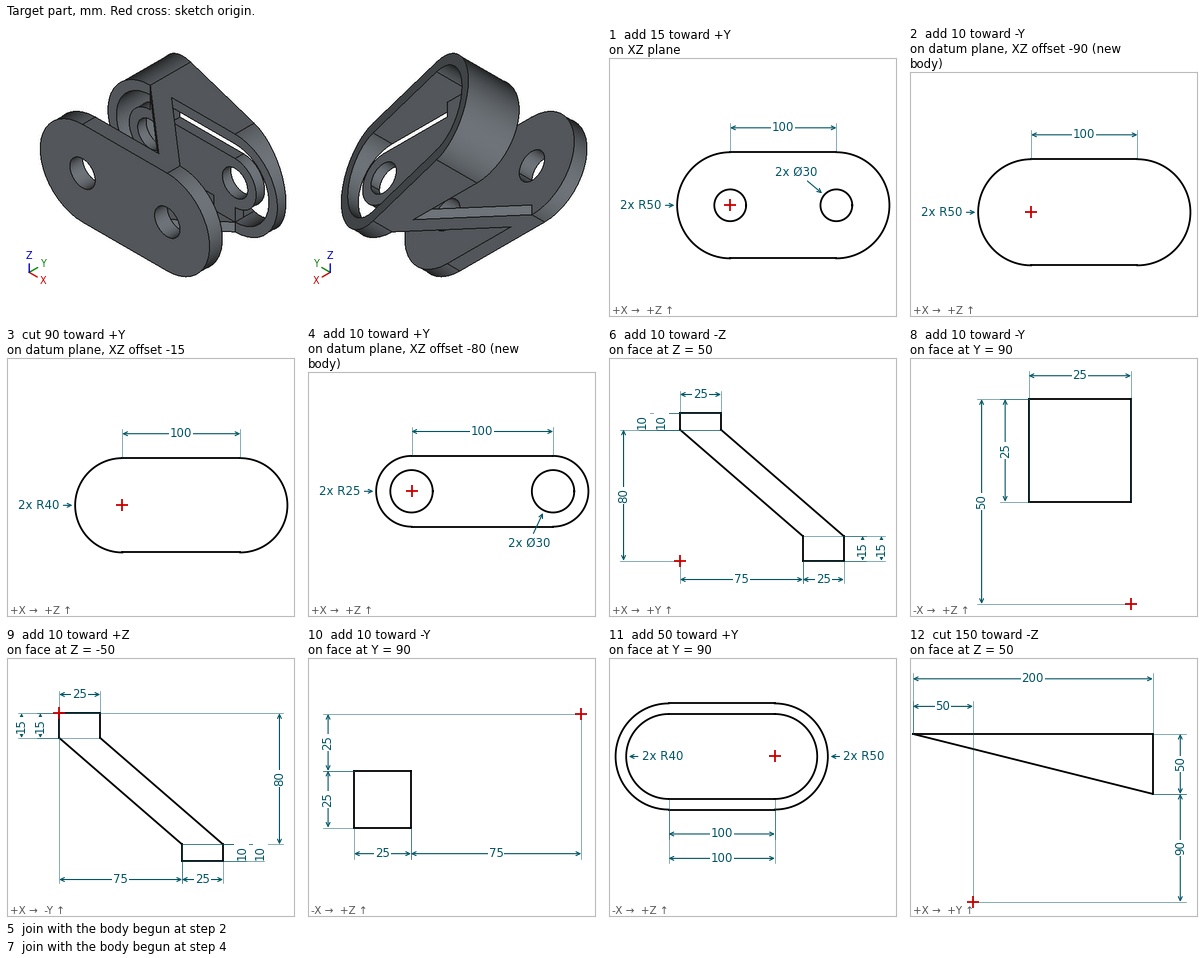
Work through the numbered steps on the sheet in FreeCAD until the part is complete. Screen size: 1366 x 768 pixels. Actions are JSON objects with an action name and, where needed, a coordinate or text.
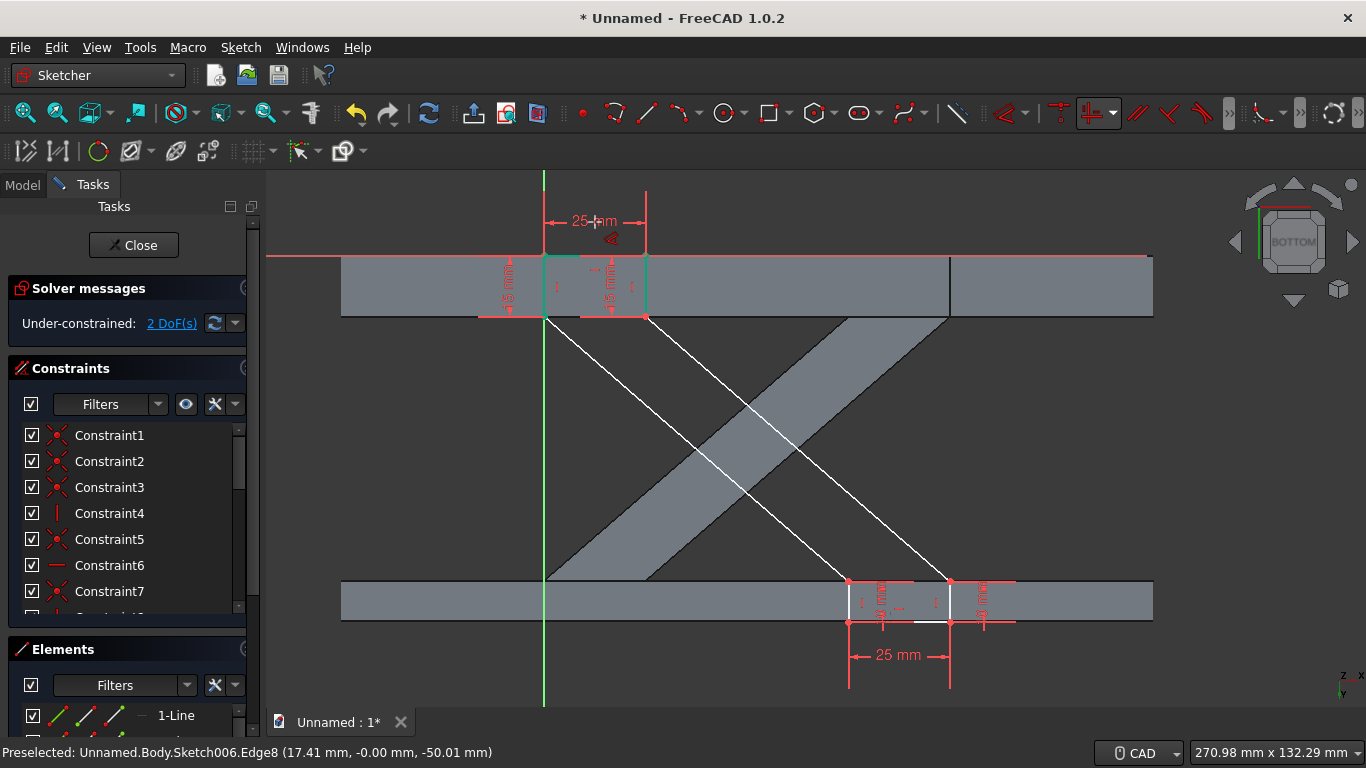
{"action": "left_click", "coordinate": [849, 582]}
{"action": "left_click", "coordinate": [696, 222]}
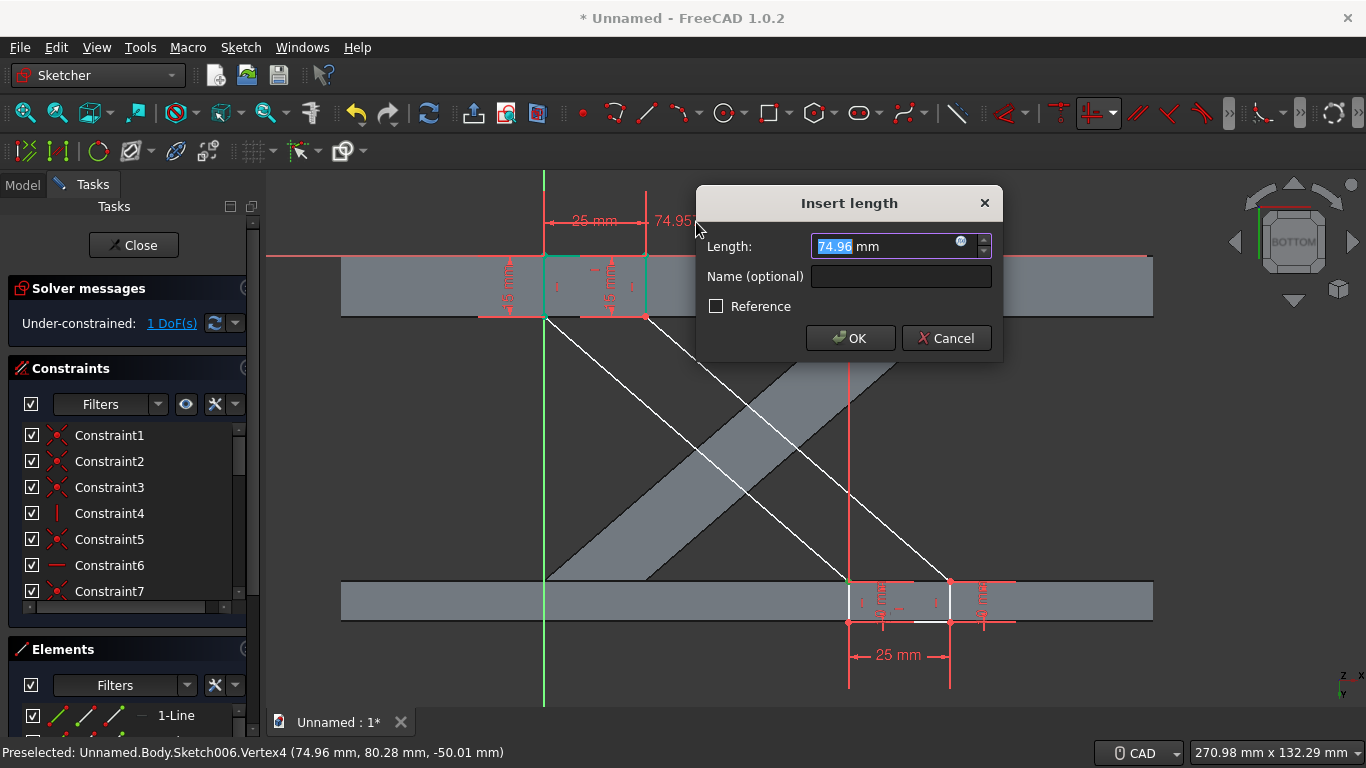
{"action": "type", "text": "75"}
{"action": "key", "text": "Return"}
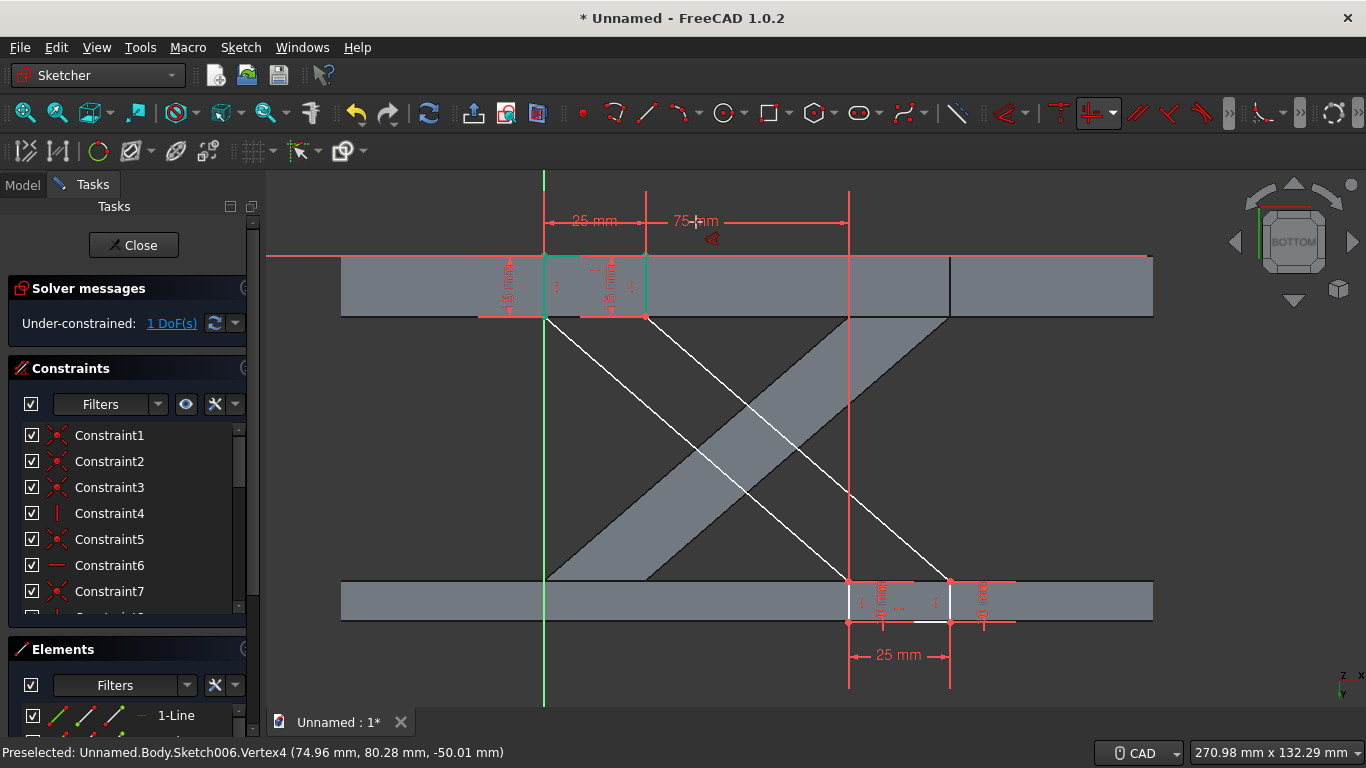
{"action": "left_click", "coordinate": [849, 582]}
{"action": "left_click", "coordinate": [510, 419]}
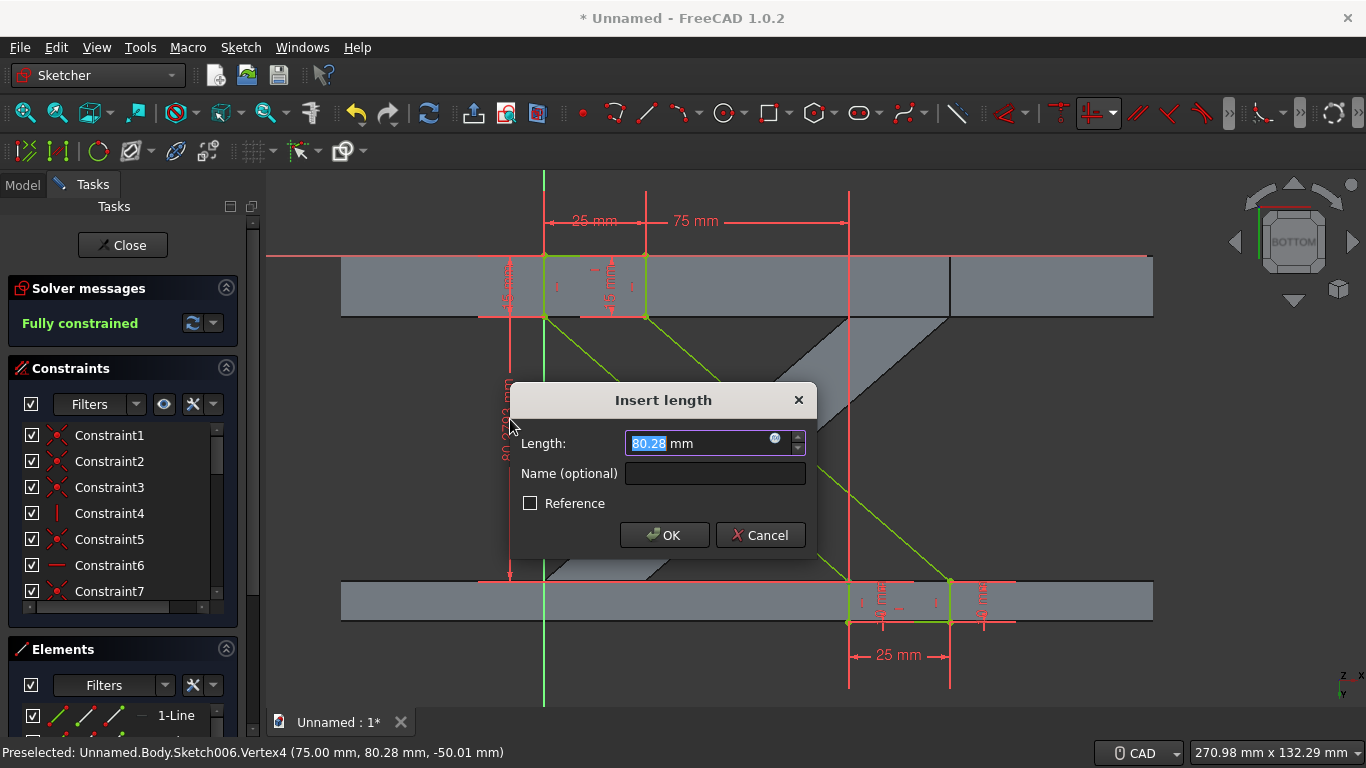
{"action": "type", "text": "80"}
{"action": "key", "text": "Return"}
{"action": "key", "text": "Escape"}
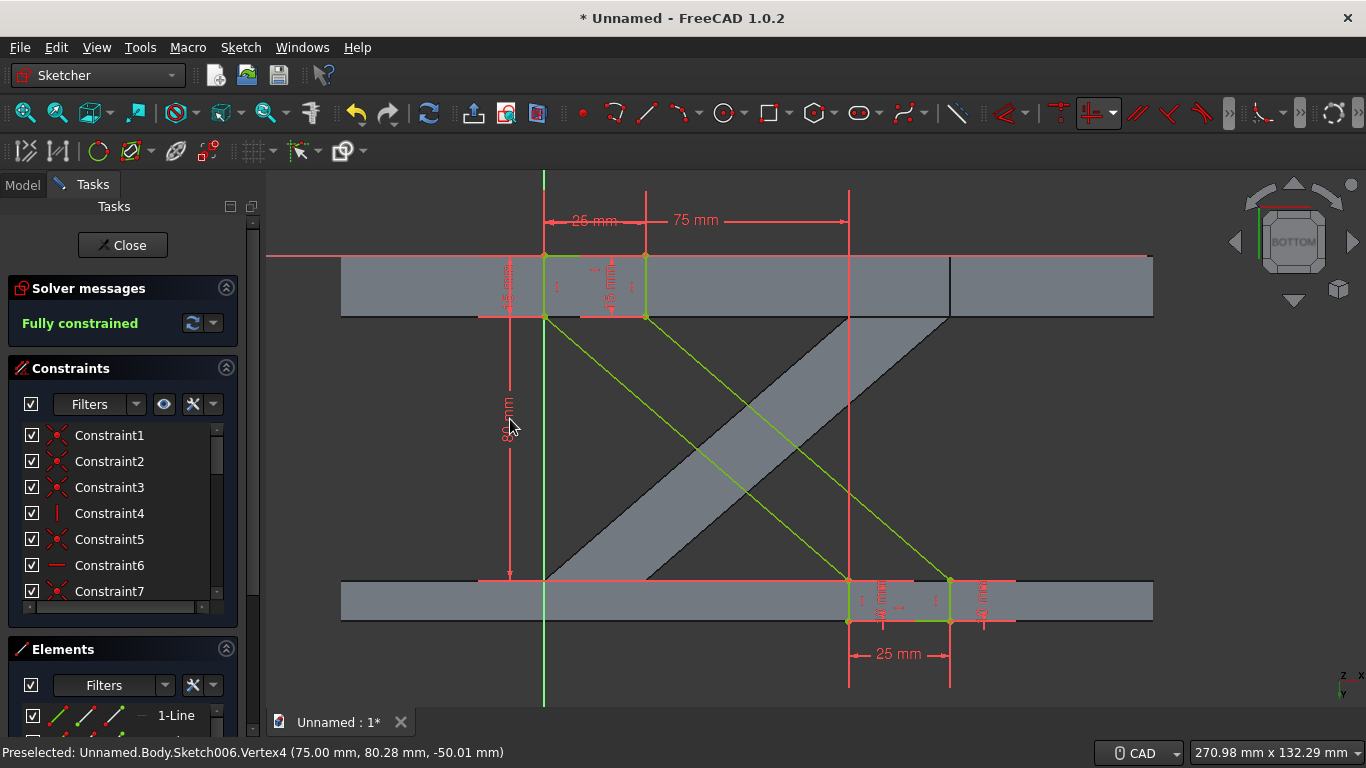
{"action": "left_click", "coordinate": [123, 245]}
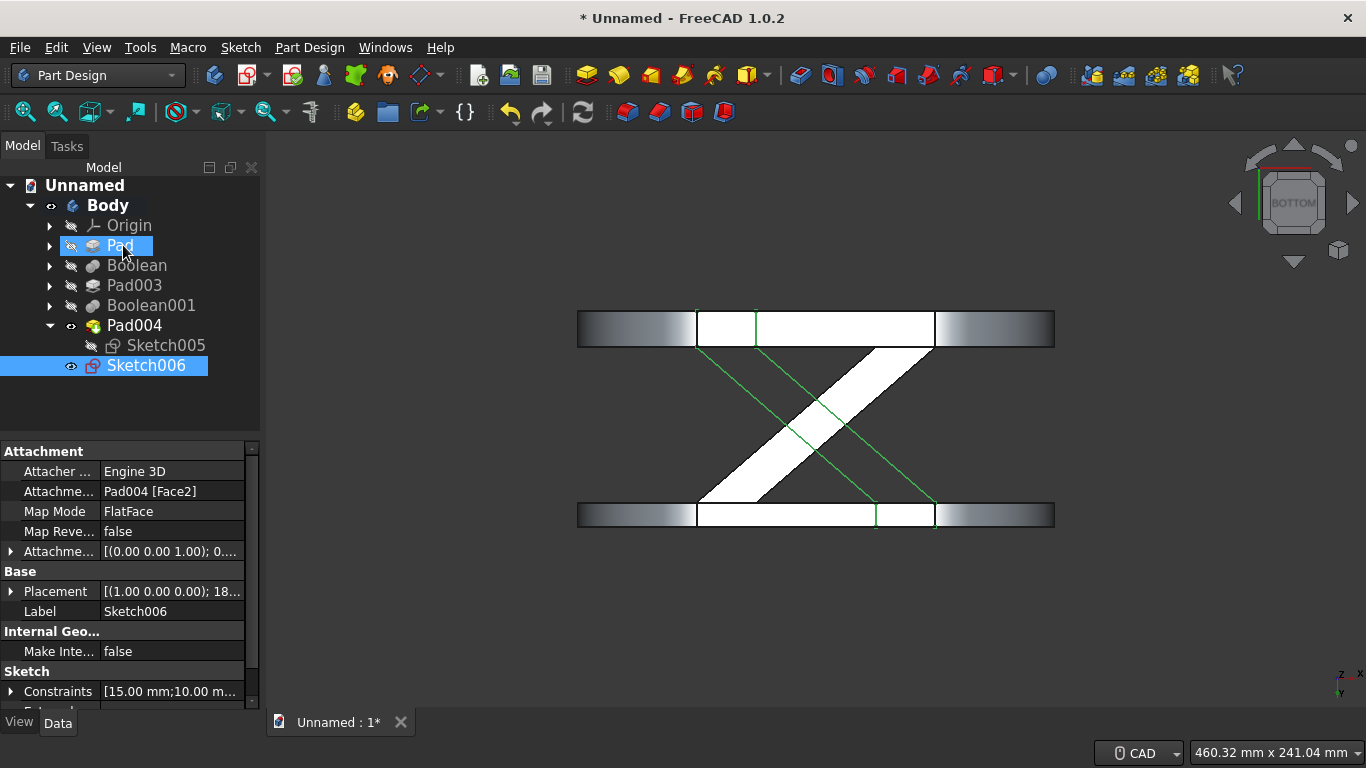
{"action": "left_click", "coordinate": [588, 76]}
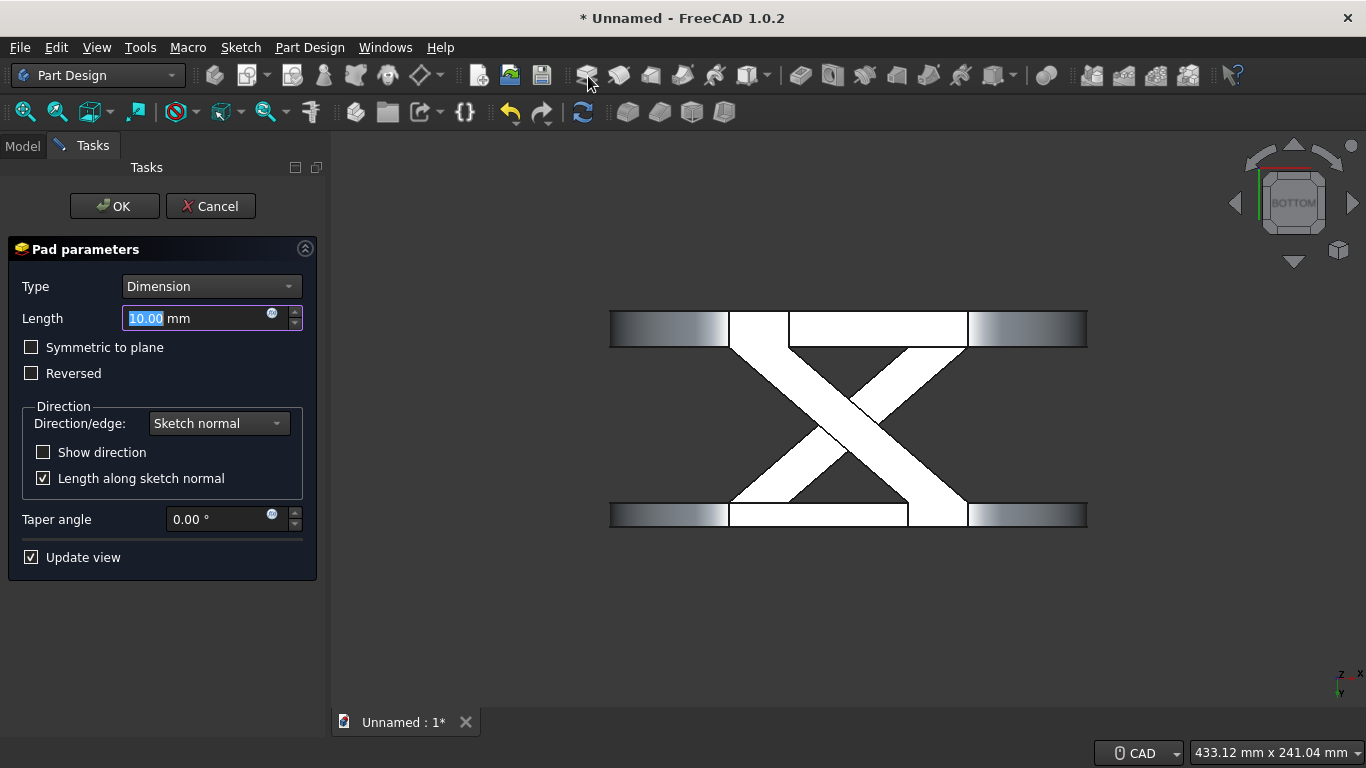
{"action": "type", "text": "10"}
{"action": "key", "text": "Tab"}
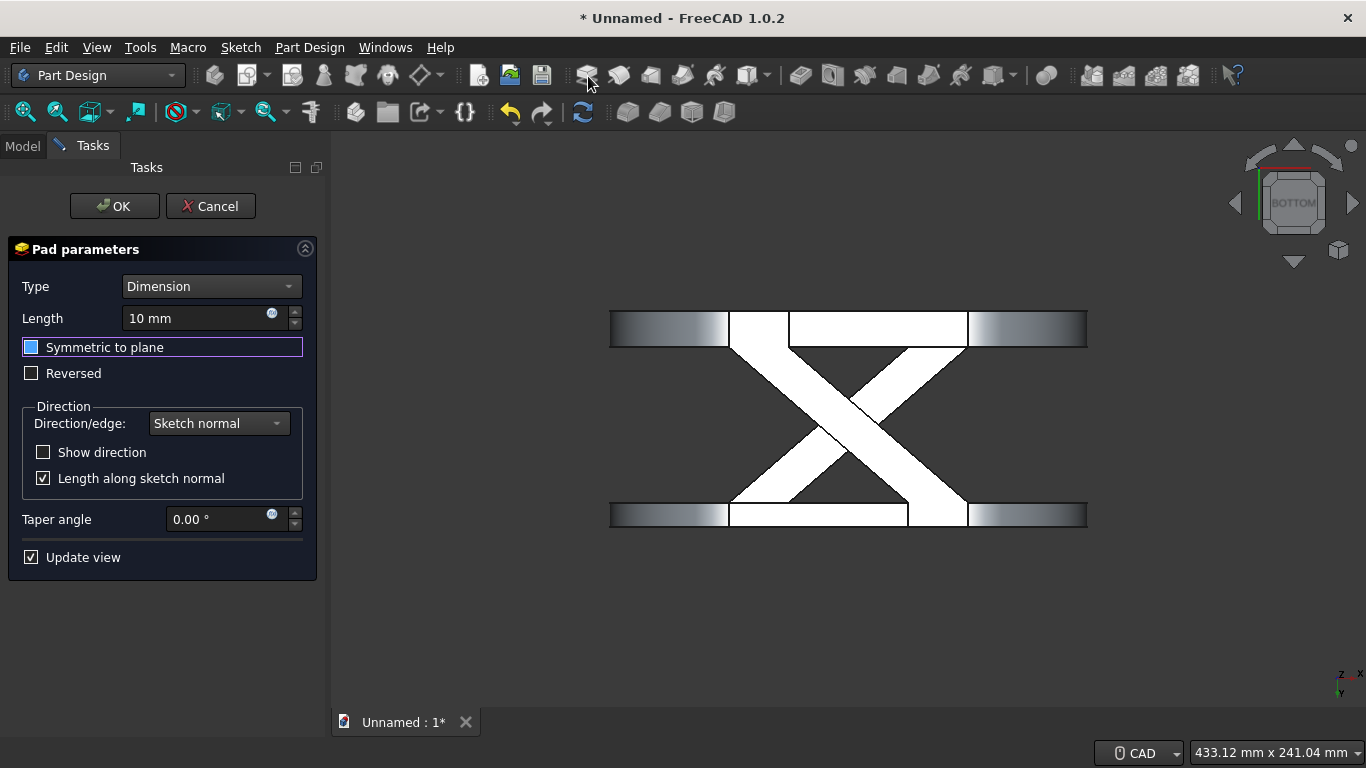
{"action": "left_click", "coordinate": [30, 373]}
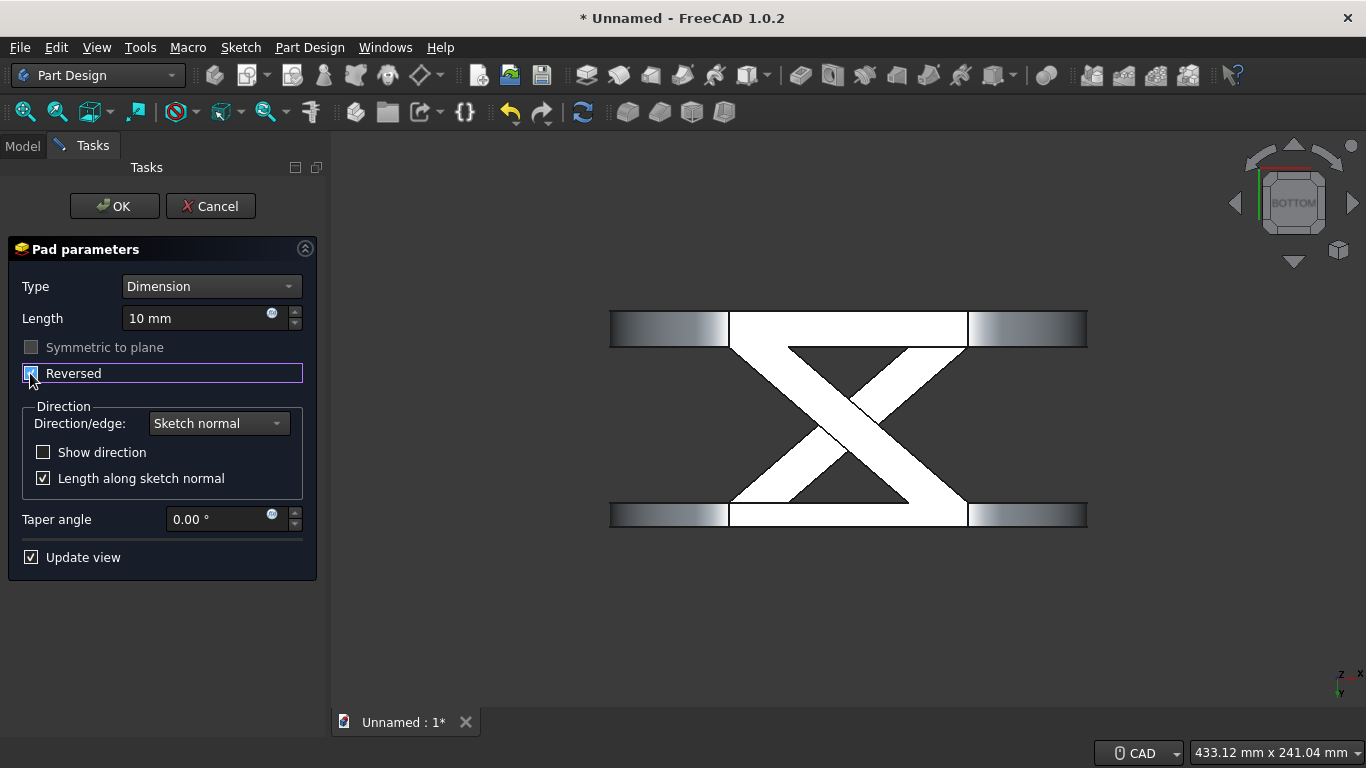
{"action": "left_click", "coordinate": [115, 206]}